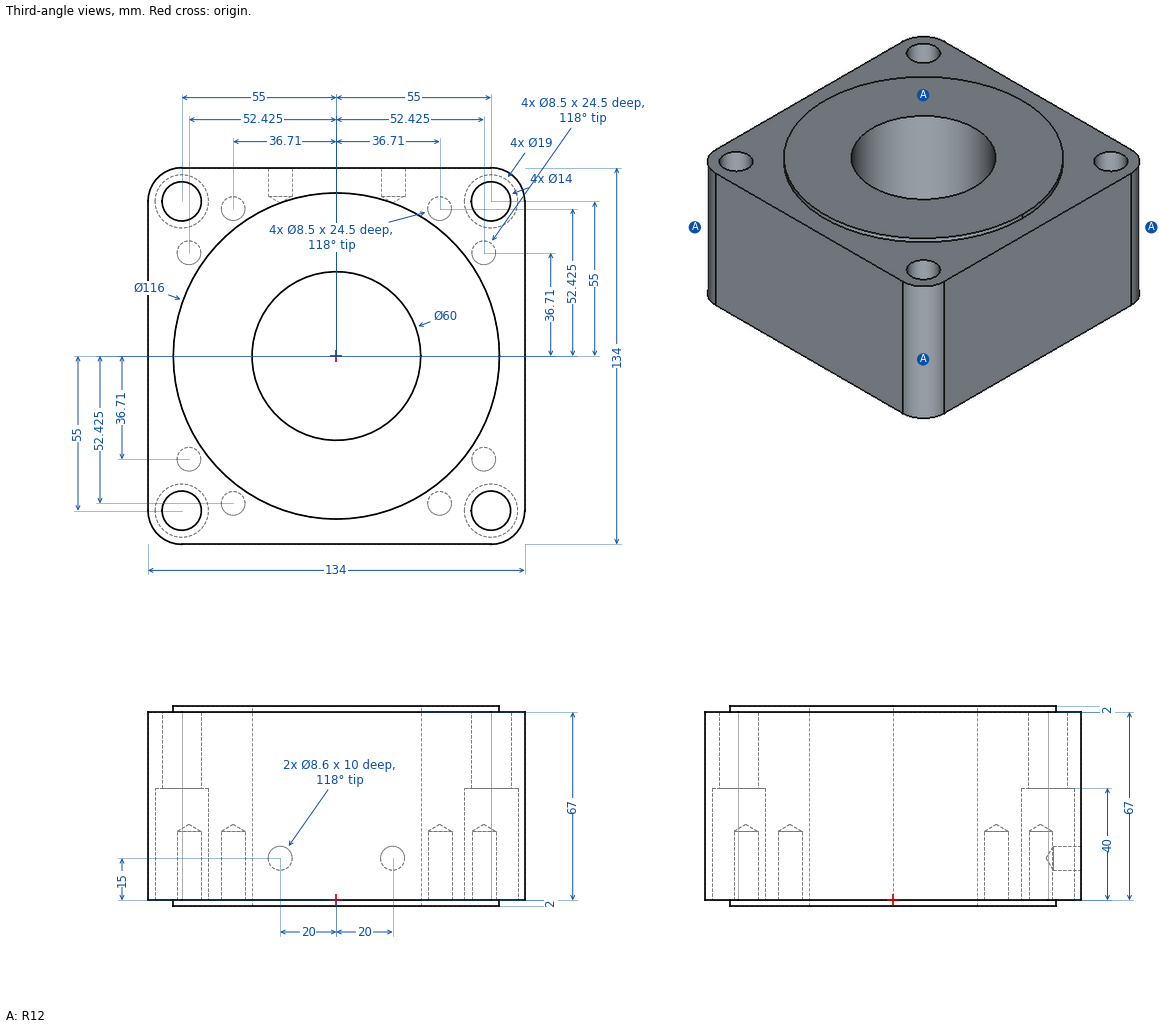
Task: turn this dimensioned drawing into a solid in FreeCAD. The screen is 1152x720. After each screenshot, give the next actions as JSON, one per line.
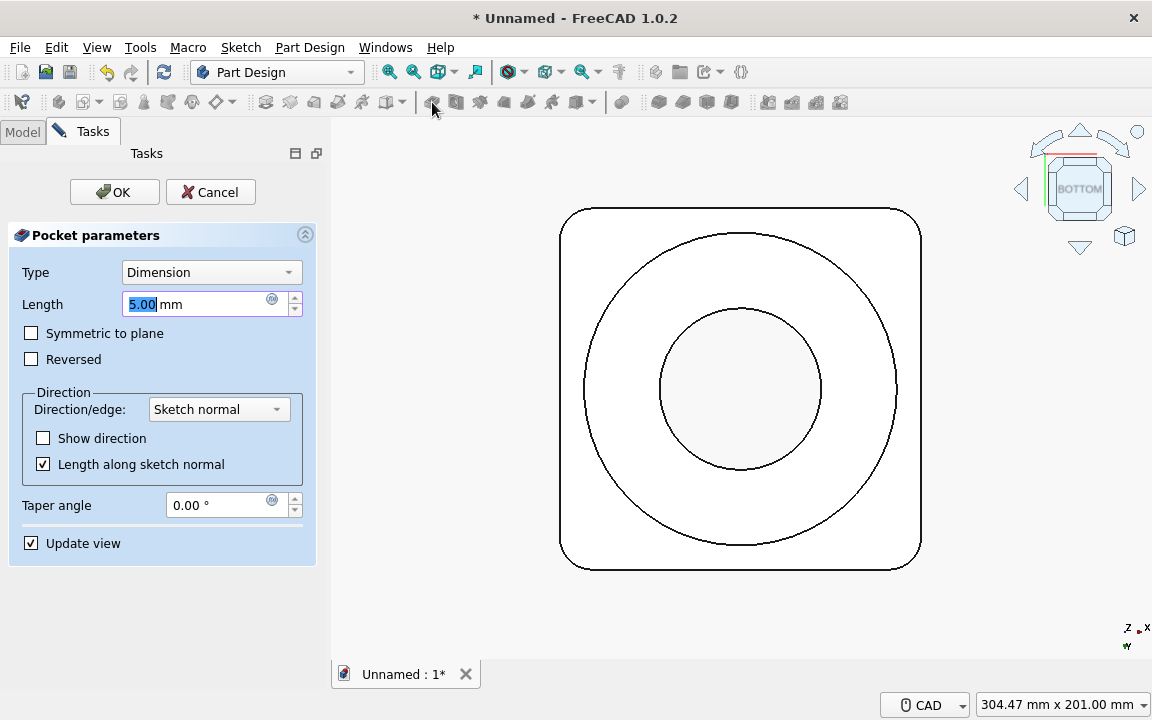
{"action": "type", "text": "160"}
{"action": "key", "text": "Tab"}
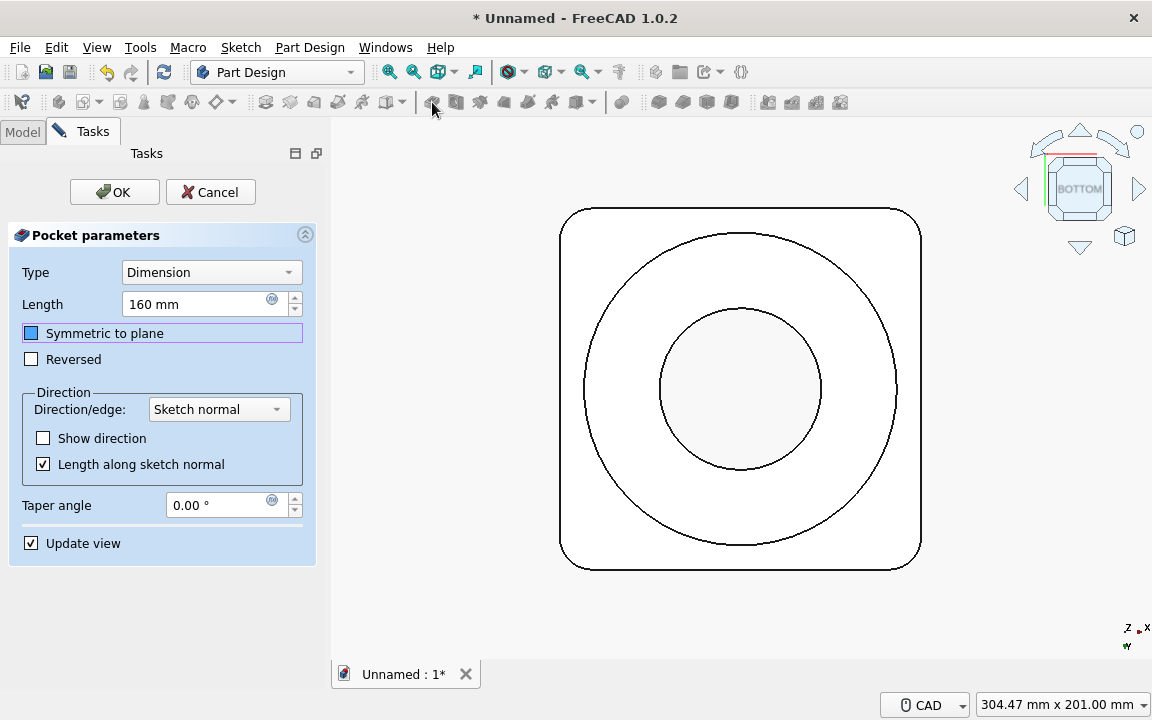
{"action": "left_click", "coordinate": [30, 359]}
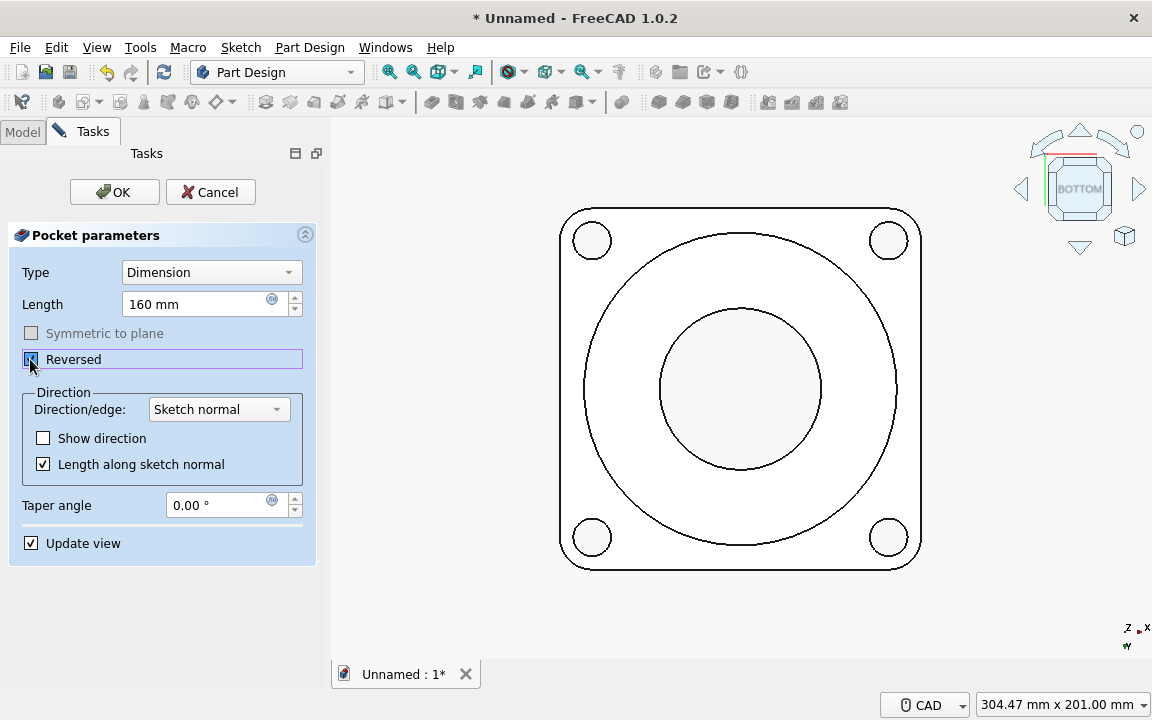
{"action": "left_click", "coordinate": [115, 192]}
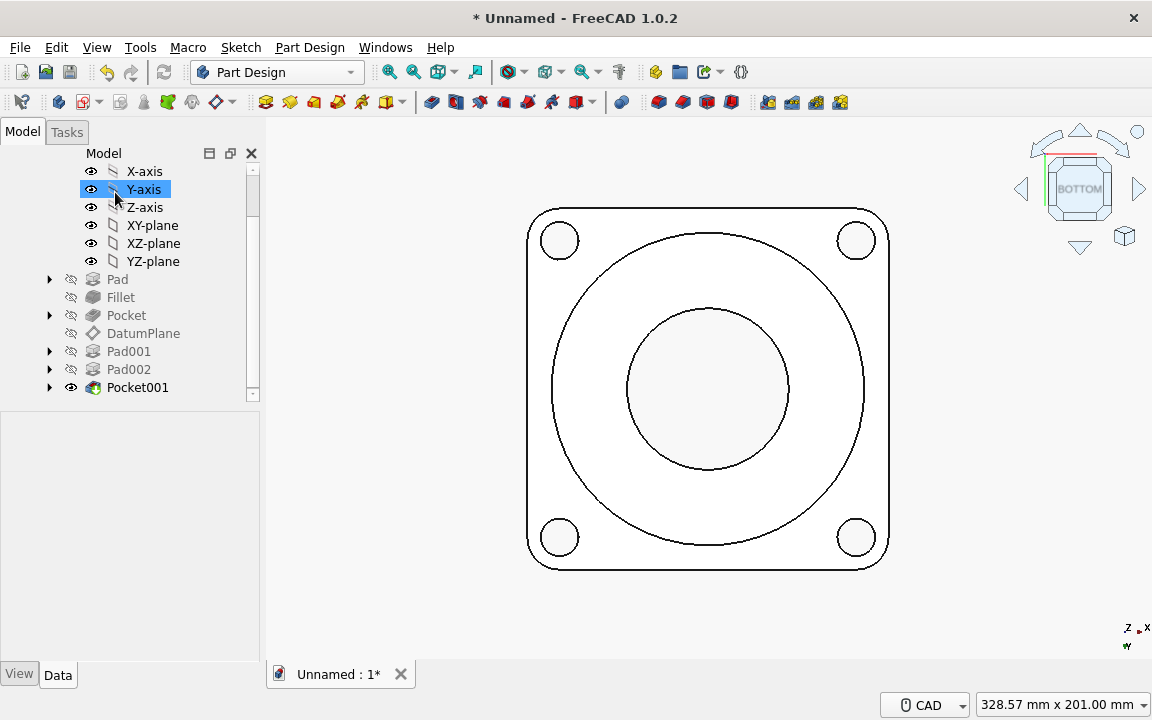
{"action": "left_click", "coordinate": [863, 491]}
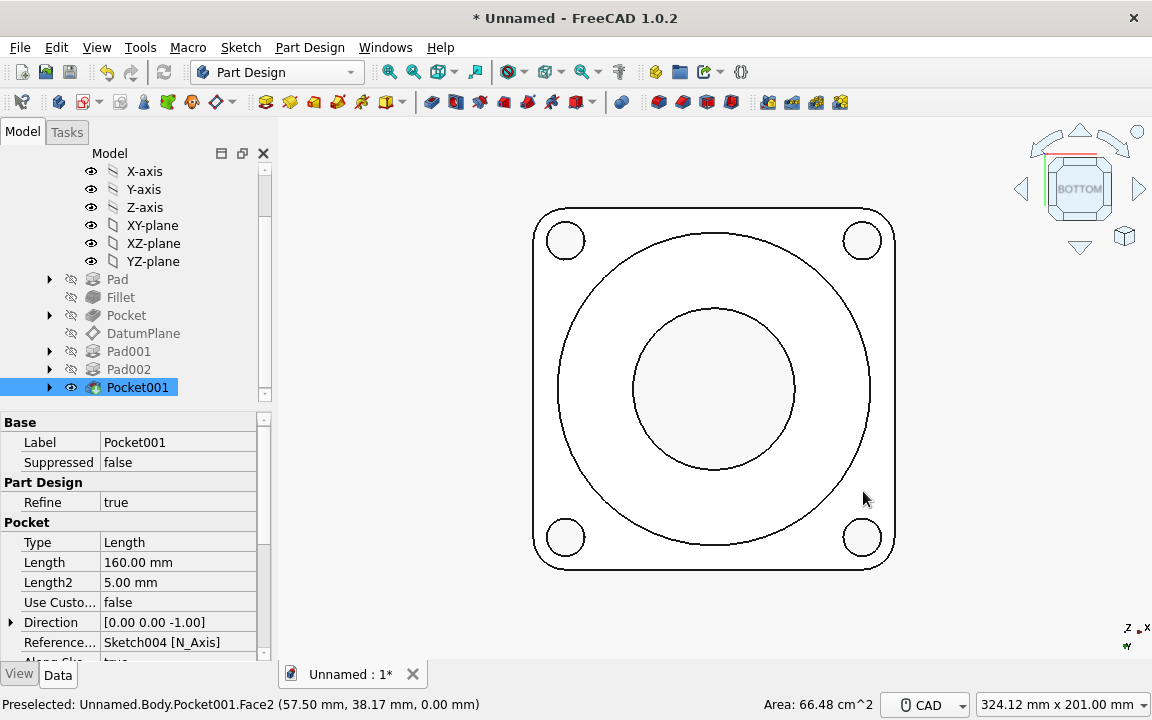
{"action": "left_click", "coordinate": [84, 102]}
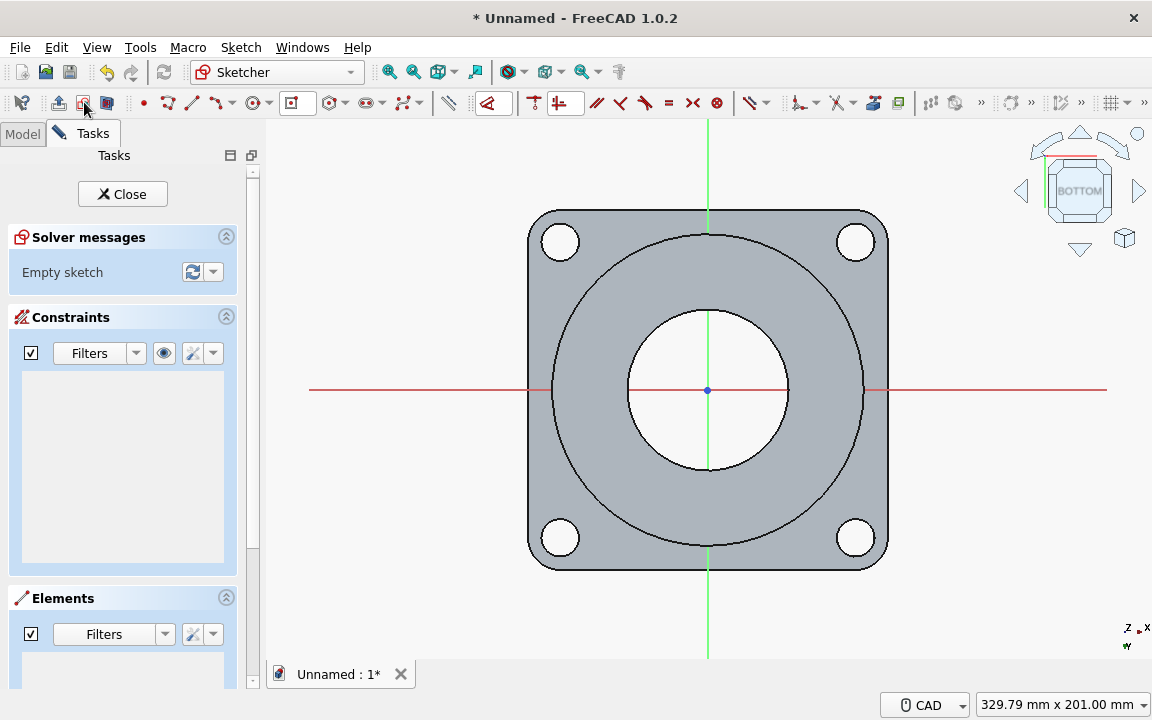
{"action": "left_click", "coordinate": [108, 104]}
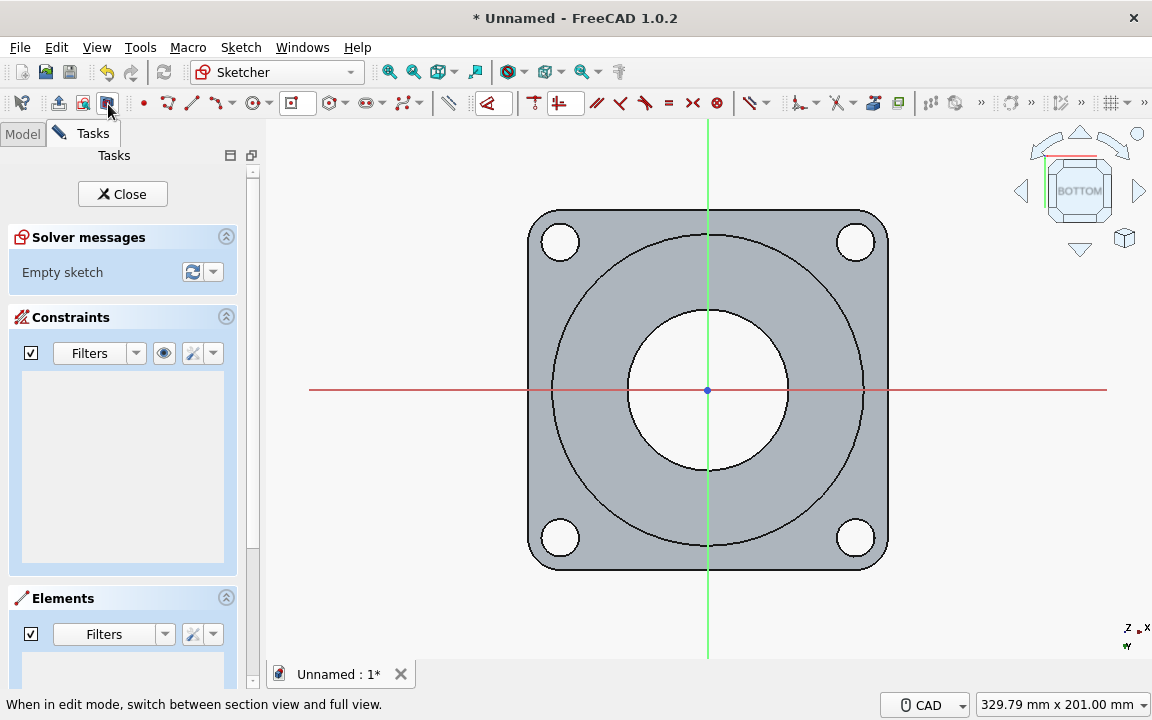
{"action": "left_click", "coordinate": [254, 104]}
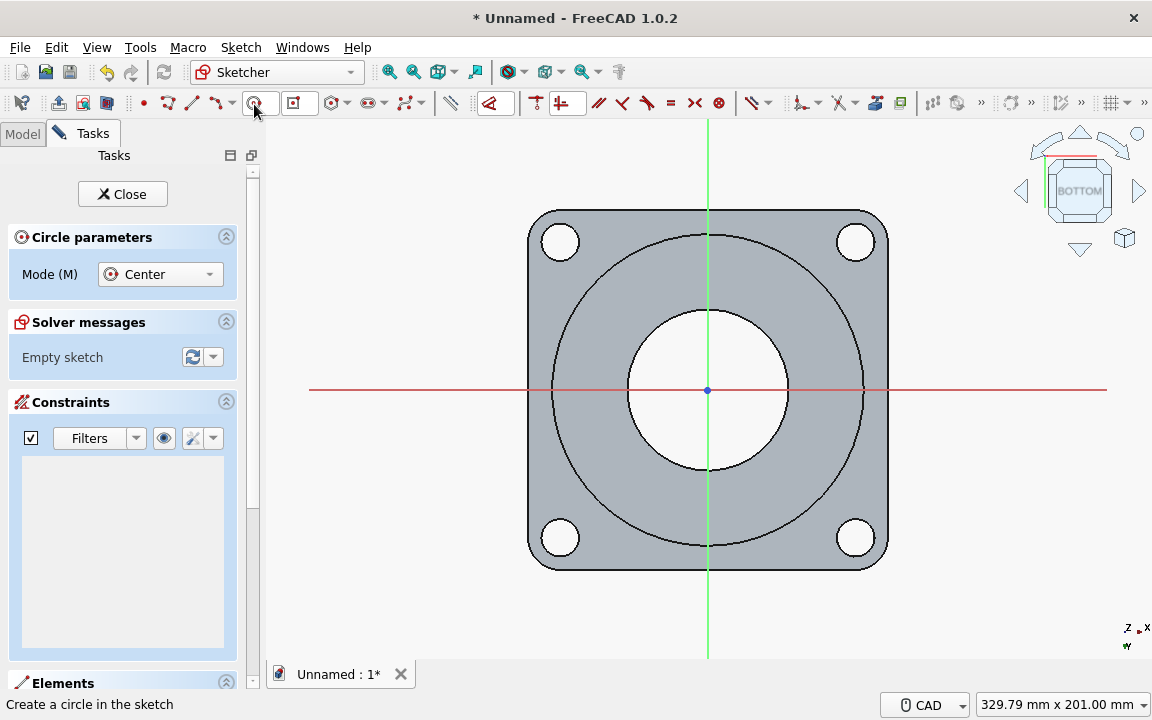
{"action": "left_click", "coordinate": [856, 538]}
{"action": "left_click", "coordinate": [874, 520]}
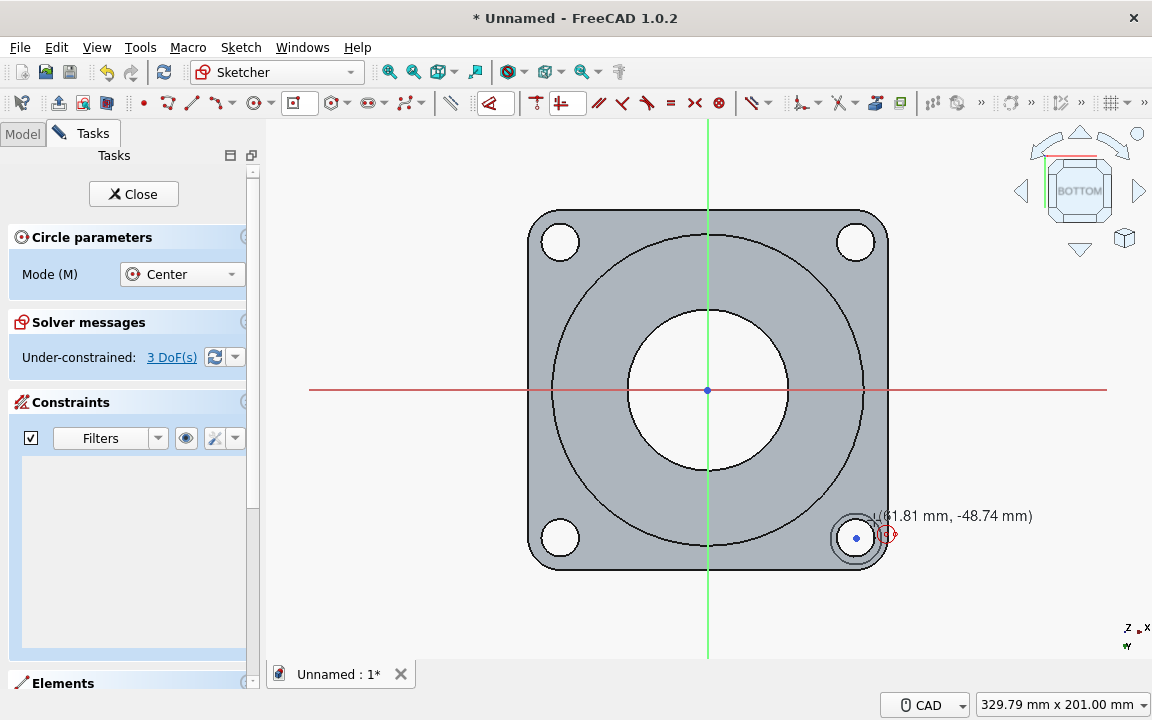
{"action": "left_click", "coordinate": [560, 538]}
{"action": "left_click", "coordinate": [578, 520]}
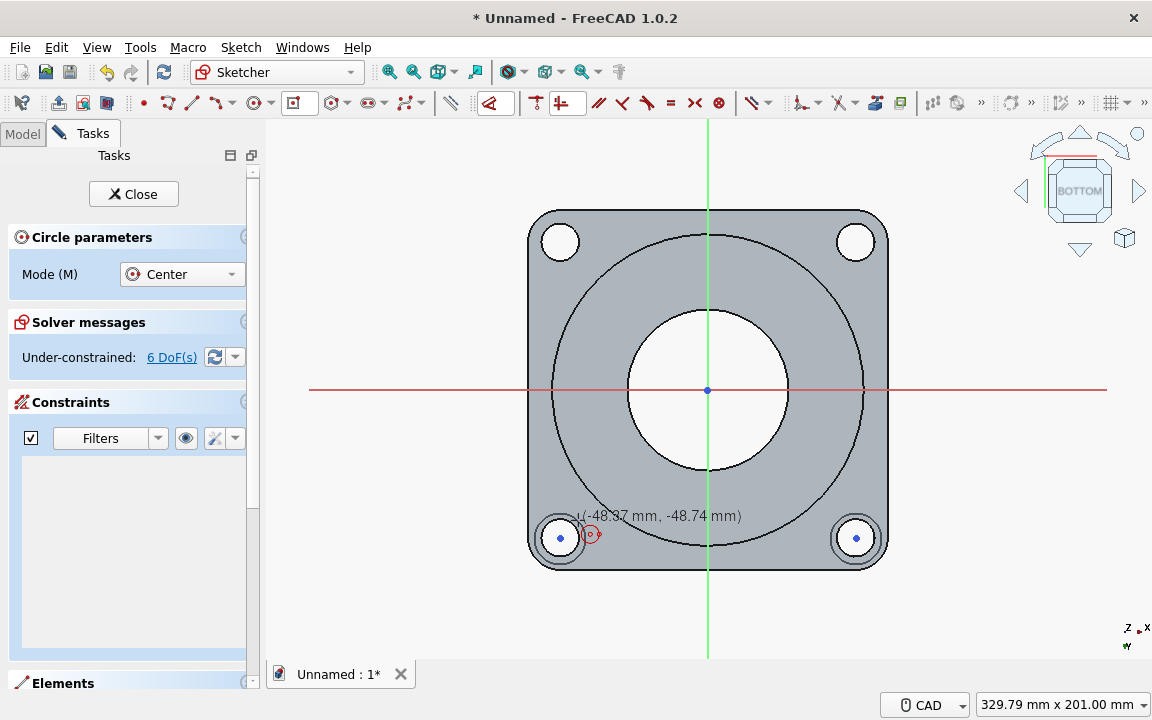
{"action": "left_click", "coordinate": [560, 242]}
{"action": "left_click", "coordinate": [578, 224]}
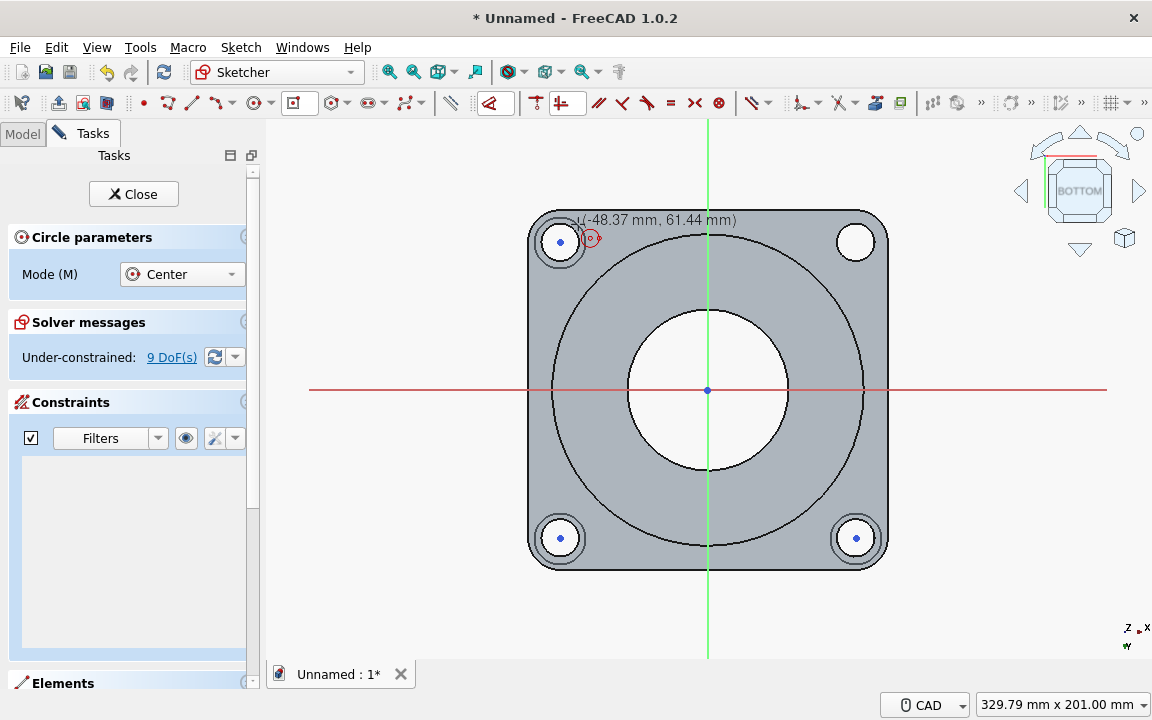
{"action": "left_click", "coordinate": [856, 242]}
{"action": "left_click", "coordinate": [874, 224]}
{"action": "key", "text": "Escape"}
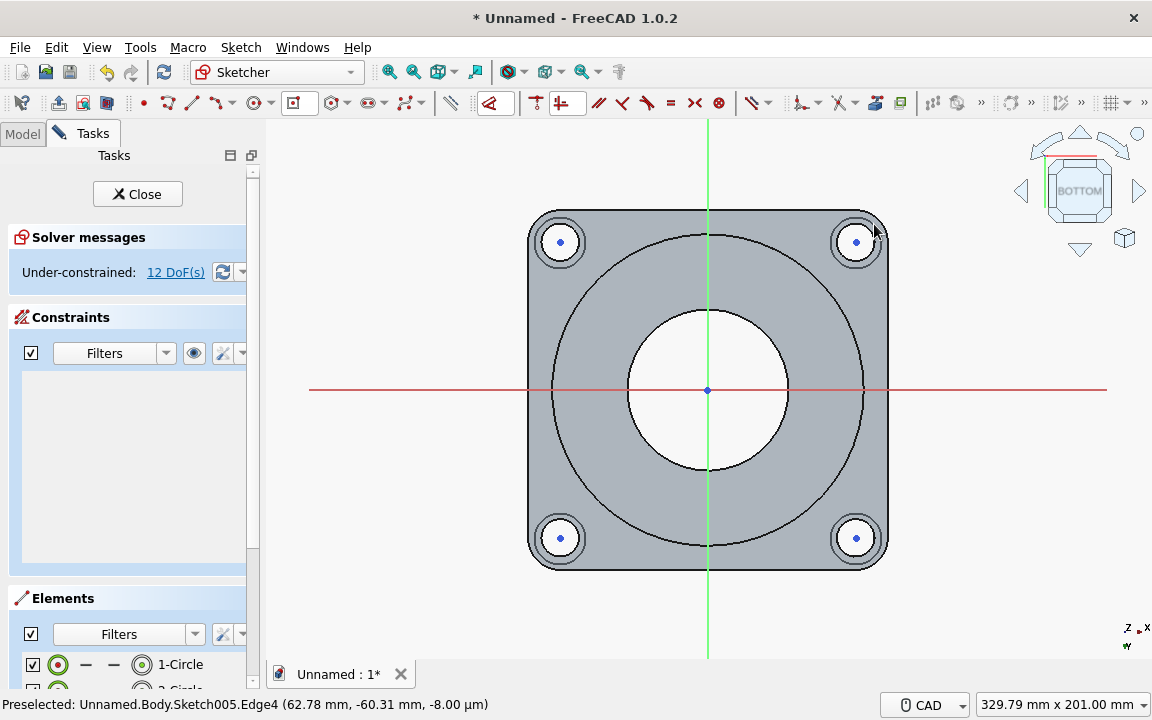
{"action": "left_click", "coordinate": [874, 521]}